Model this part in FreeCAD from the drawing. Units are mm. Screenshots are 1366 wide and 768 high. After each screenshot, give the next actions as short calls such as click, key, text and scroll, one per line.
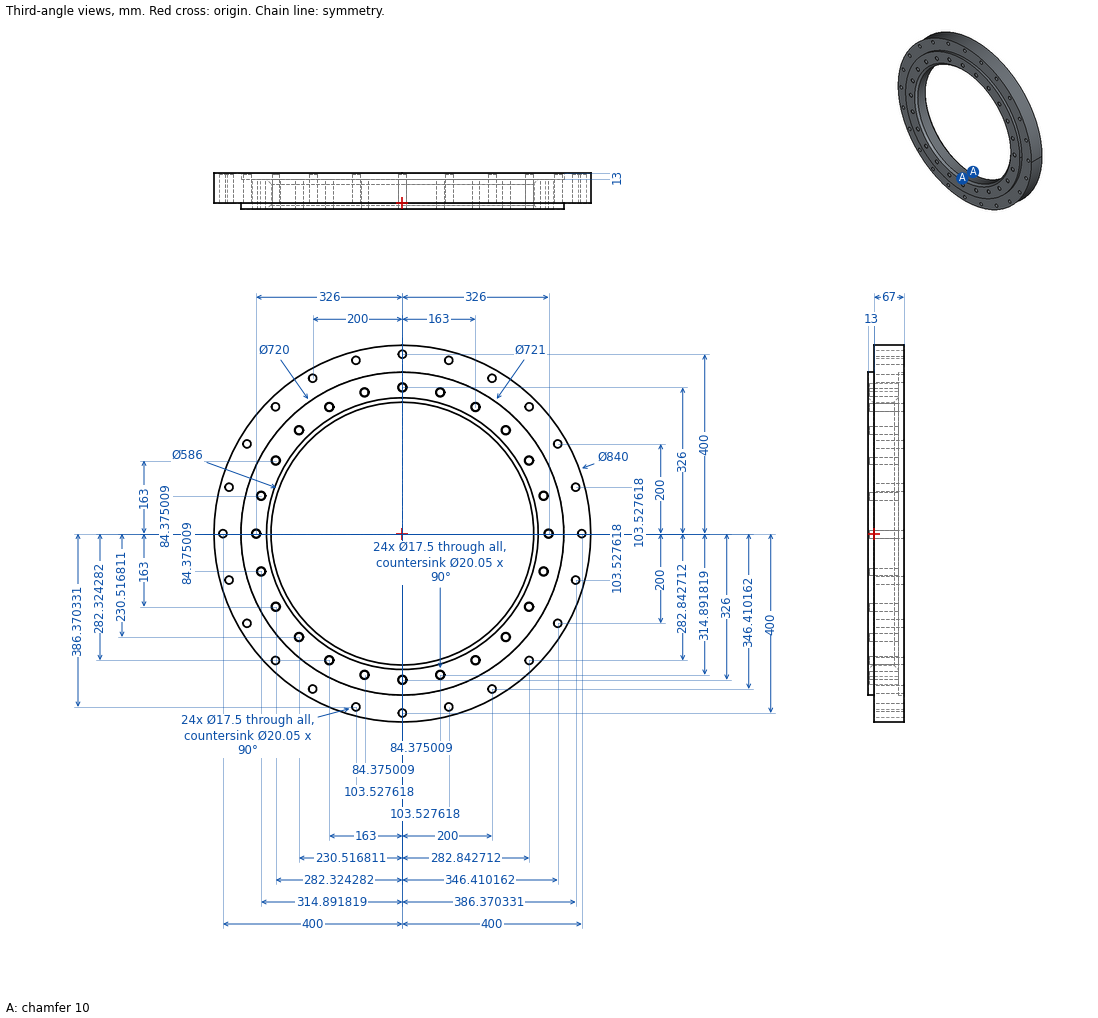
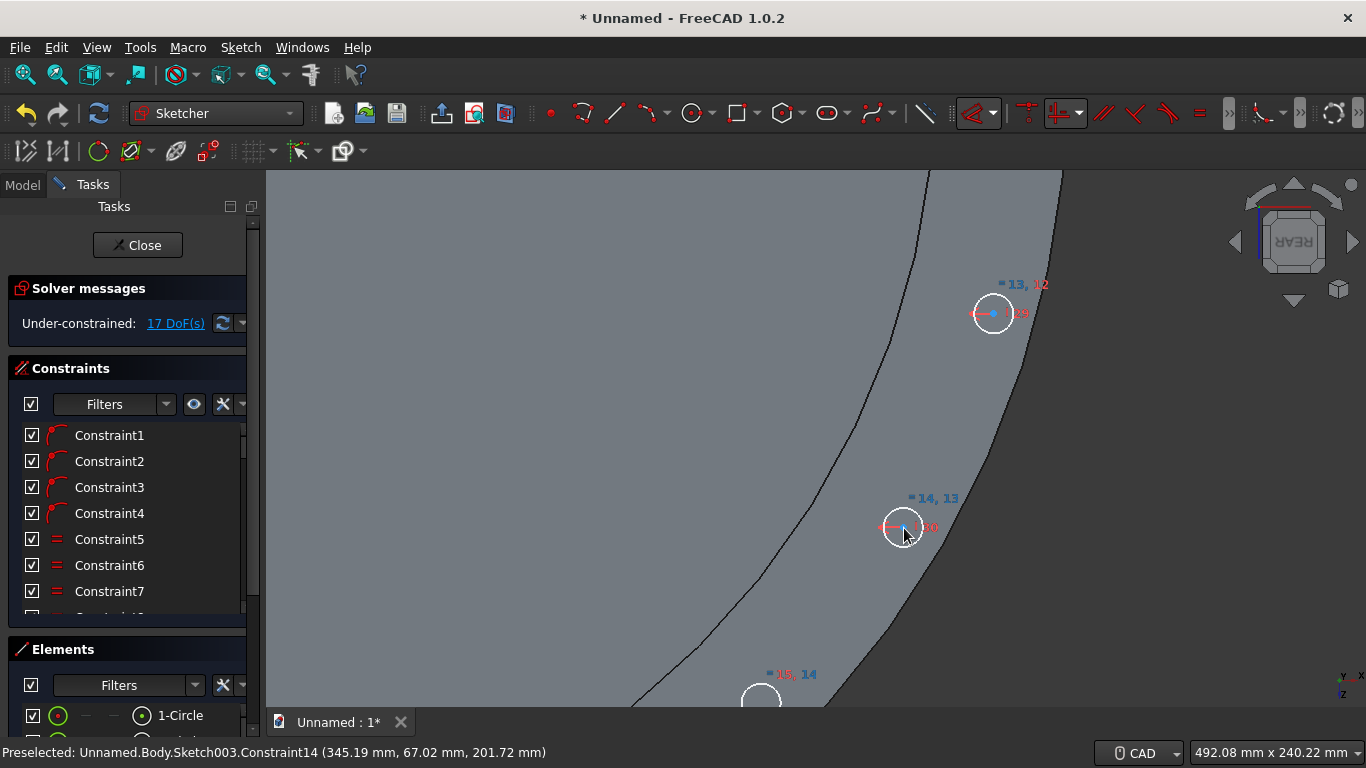
click(903, 527)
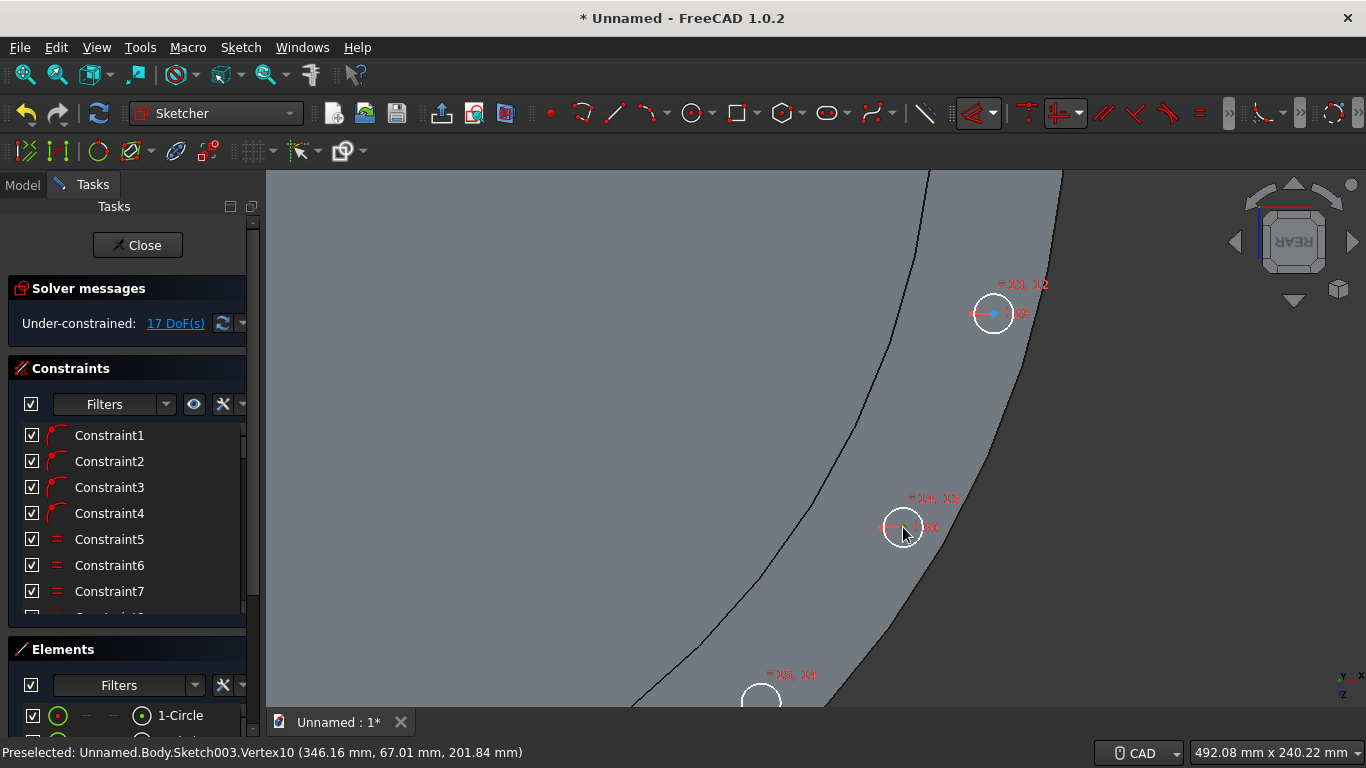
key(i)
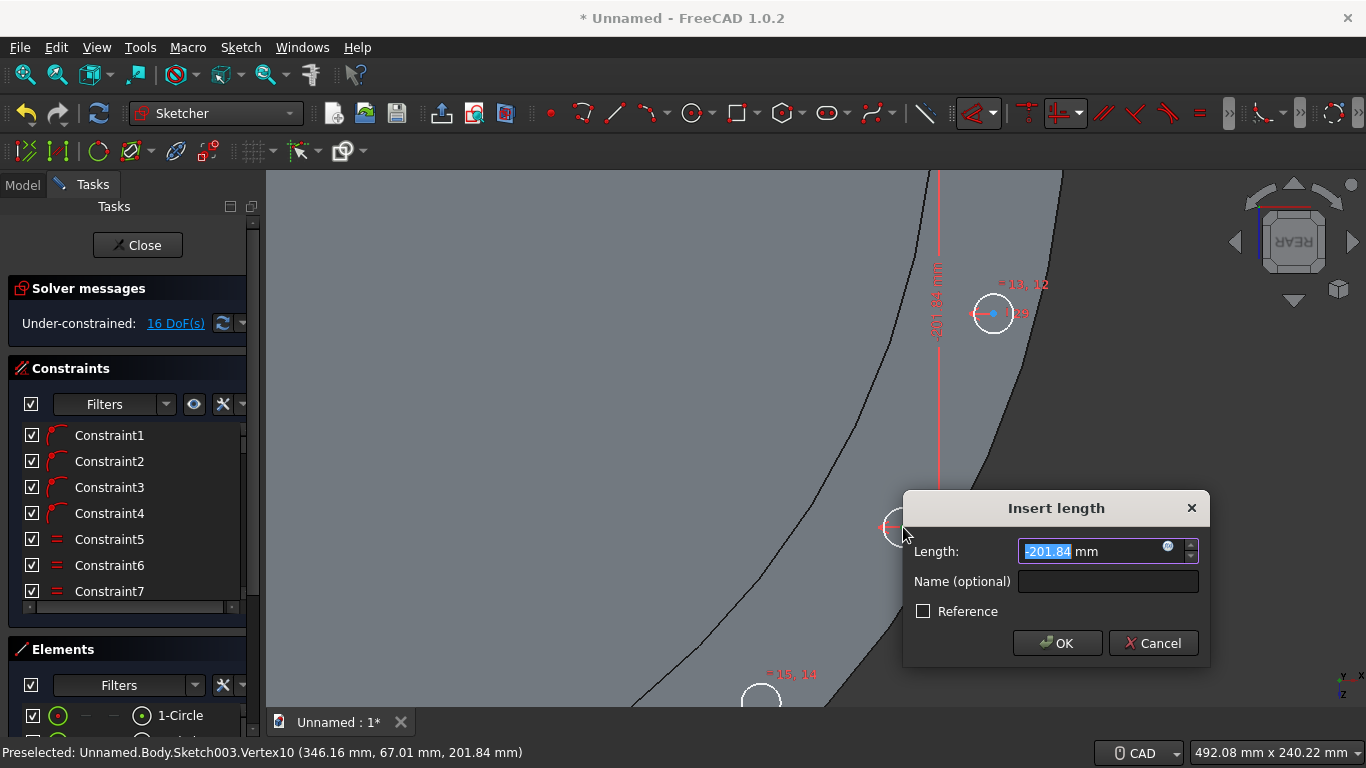
text(-200)
key(Return)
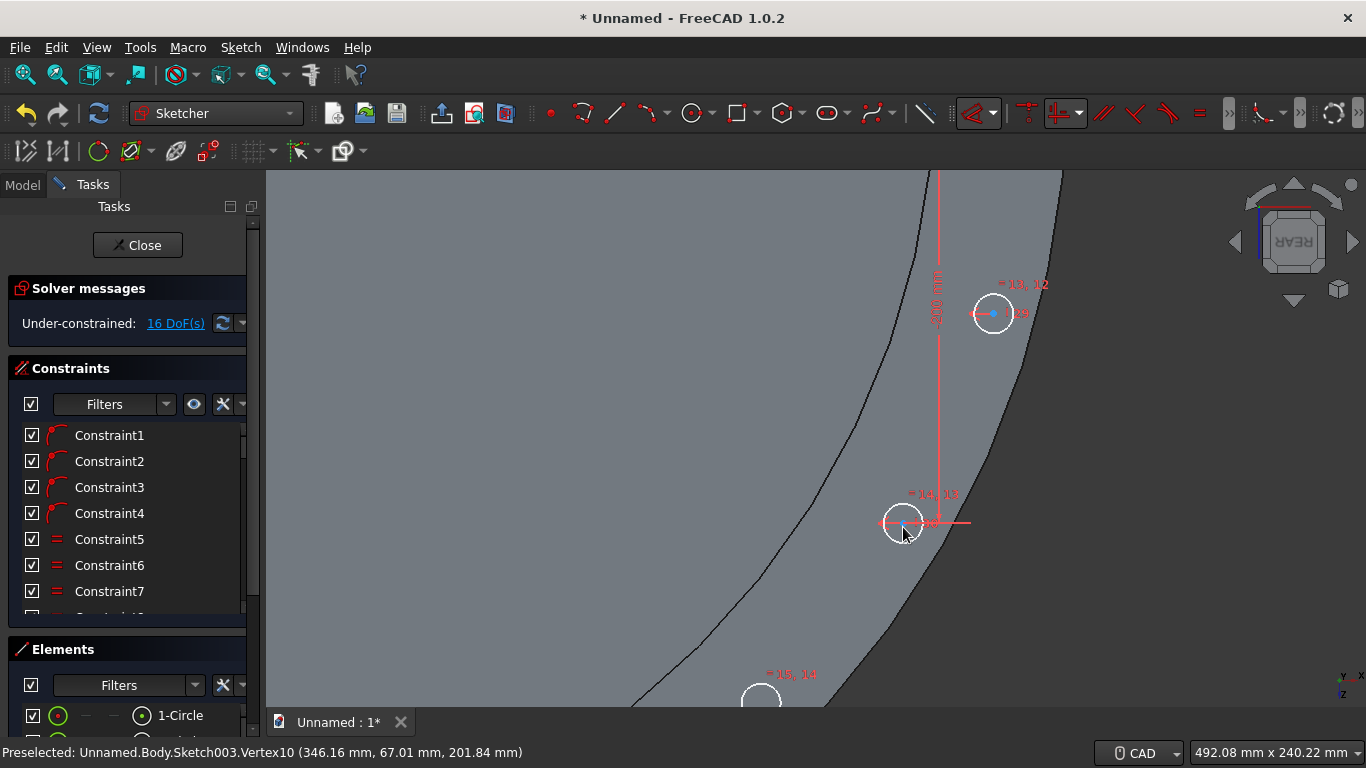
scroll(904, 530, down, 8)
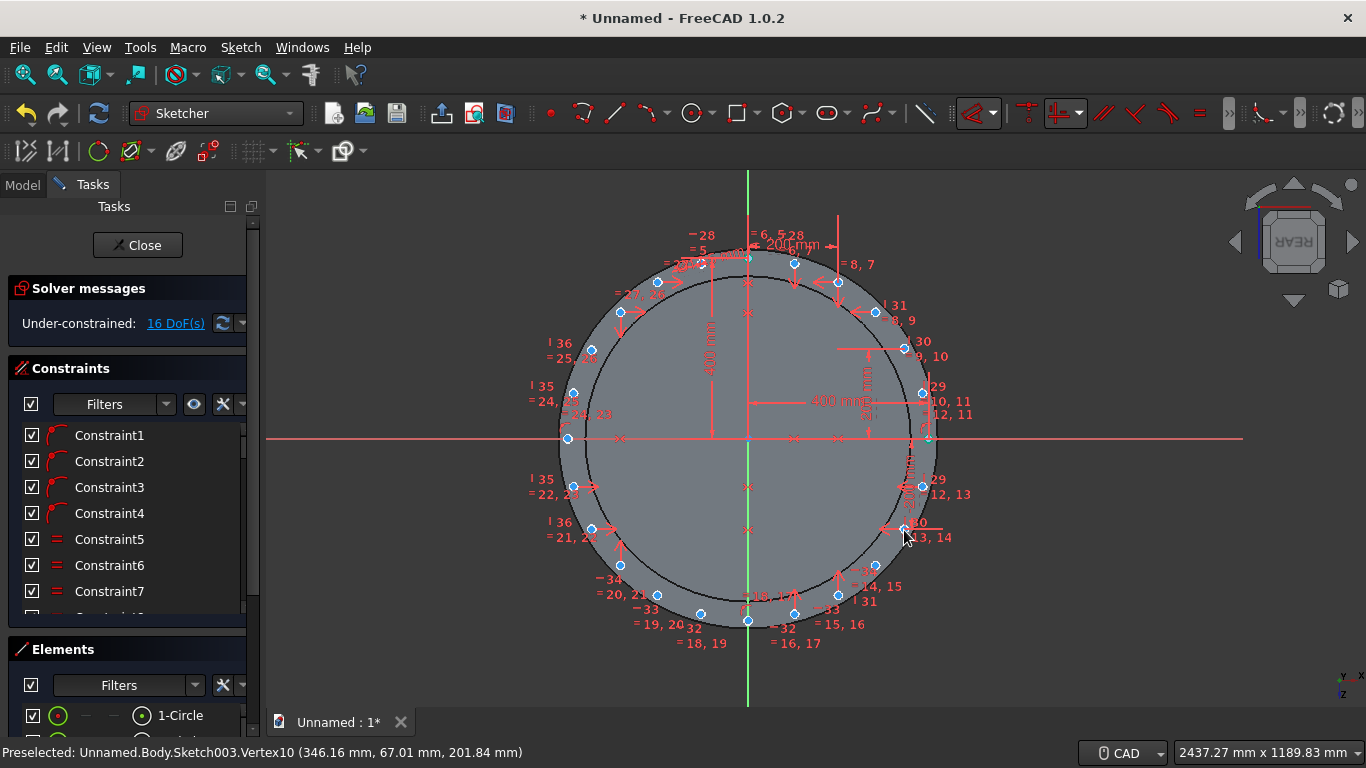
click(748, 621)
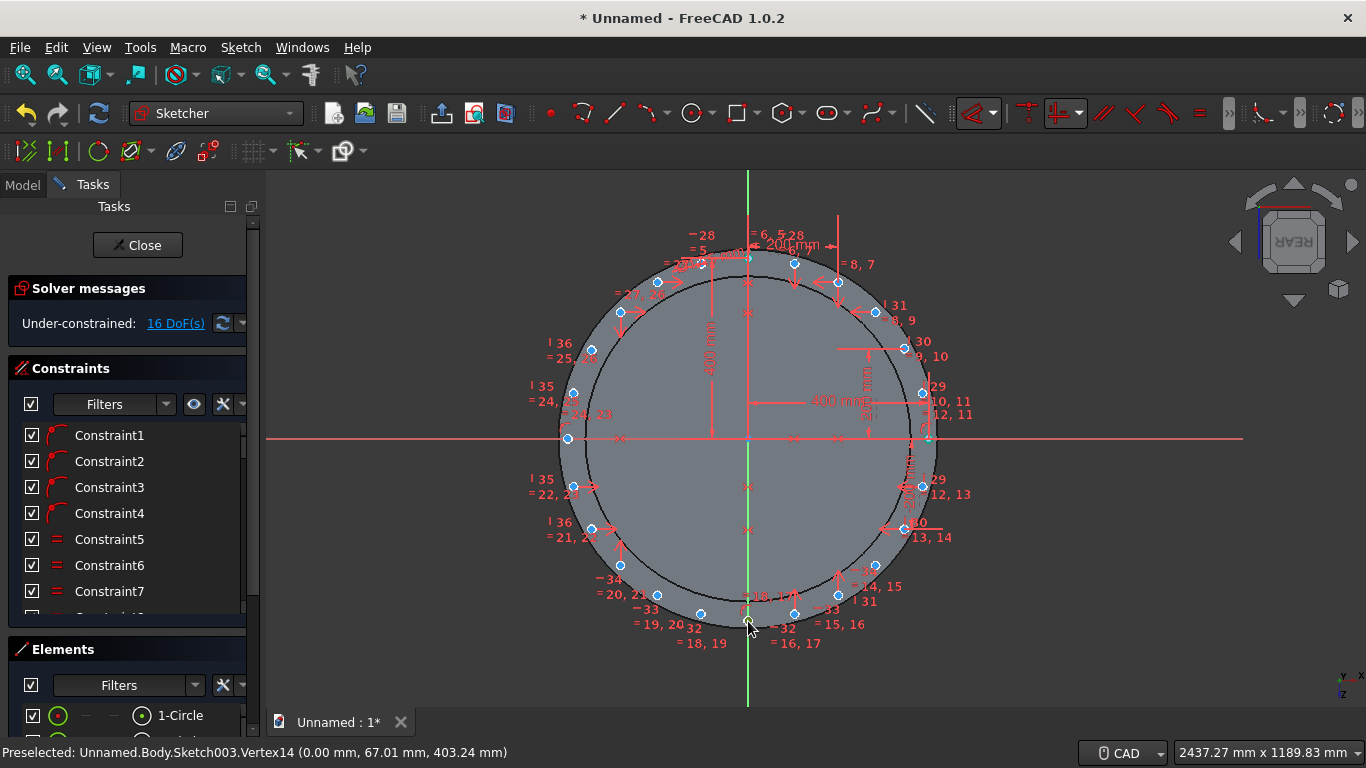
key(i)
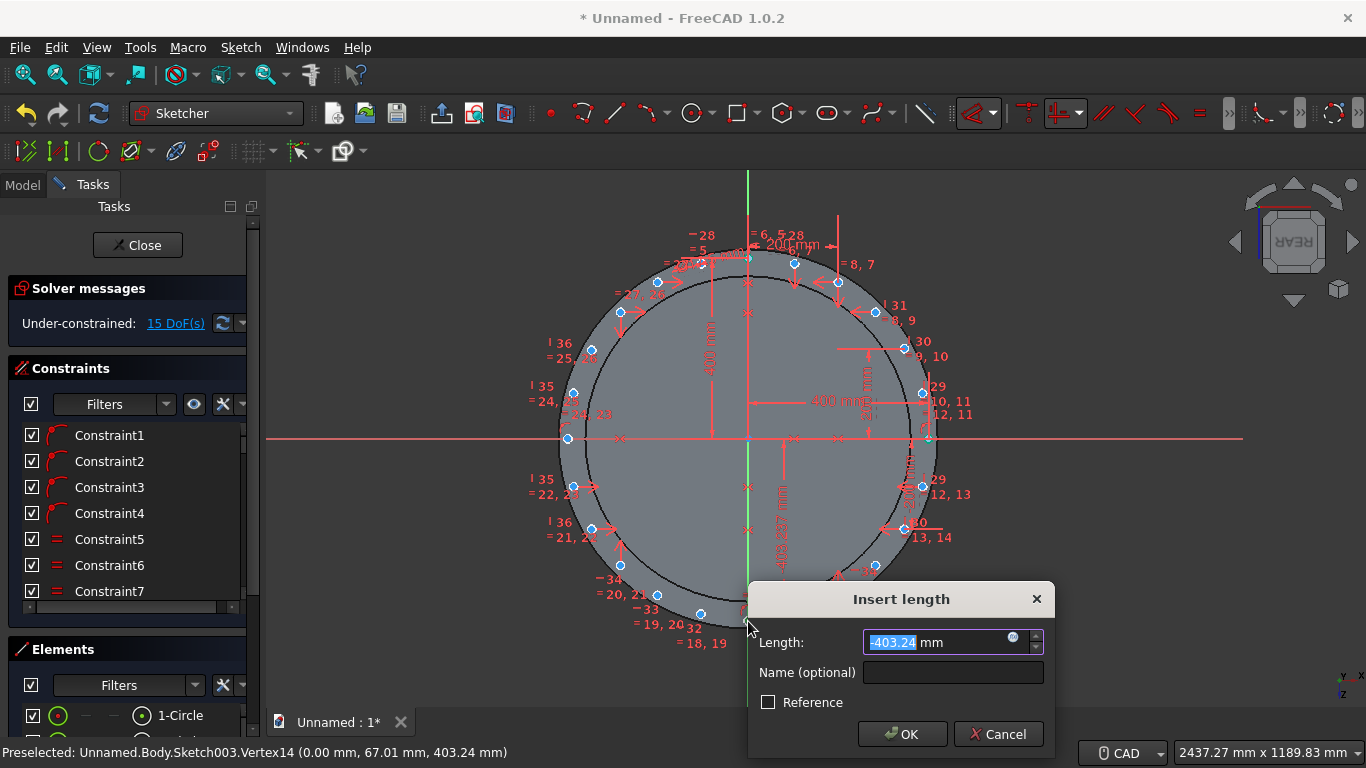
text(-400)
key(Return)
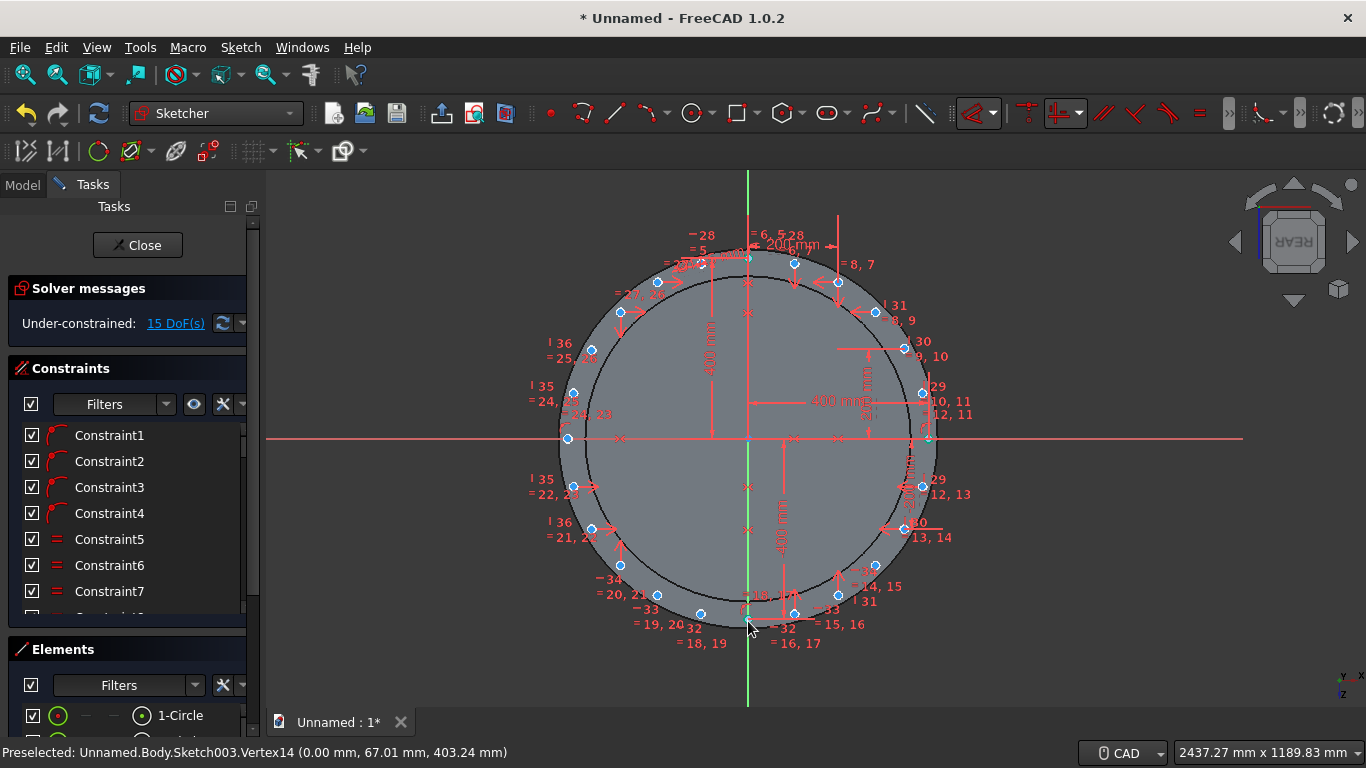
click(657, 595)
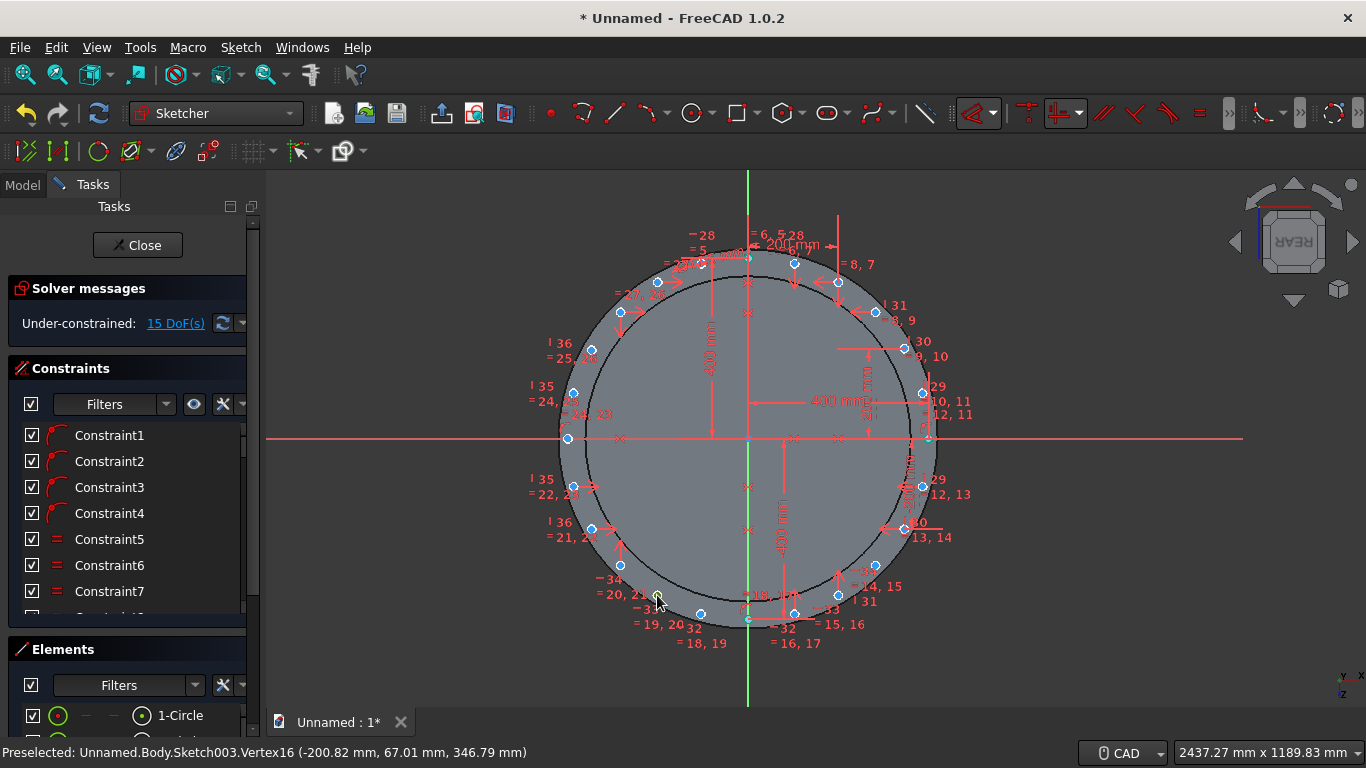
key(l)